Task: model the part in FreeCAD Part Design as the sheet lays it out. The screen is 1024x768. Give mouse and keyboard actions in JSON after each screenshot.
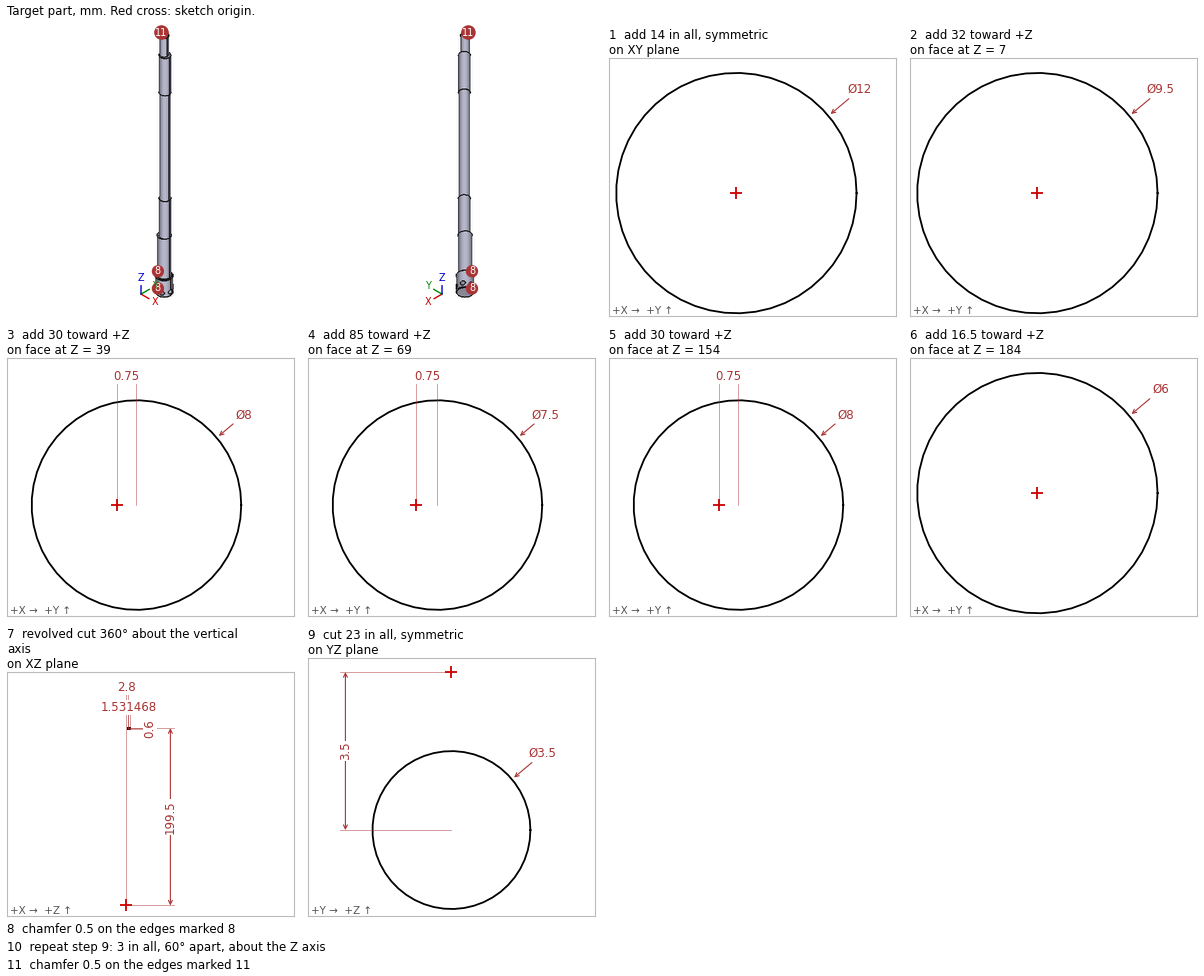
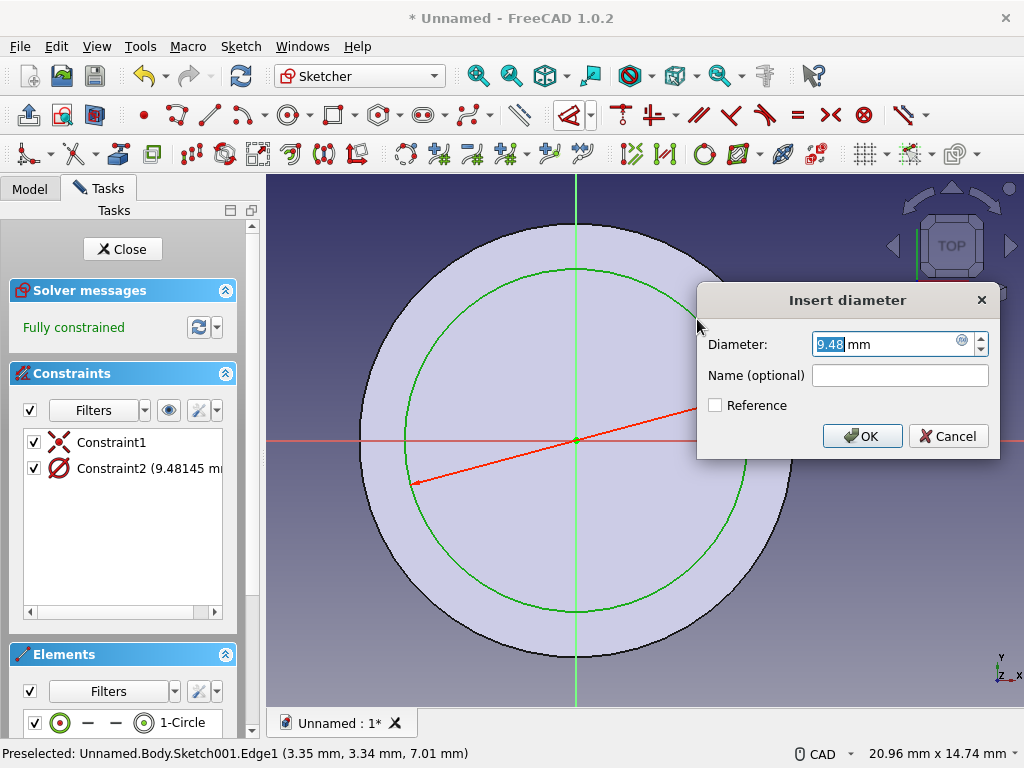
{"action": "type", "text": "9.5"}
{"action": "key", "text": "Return"}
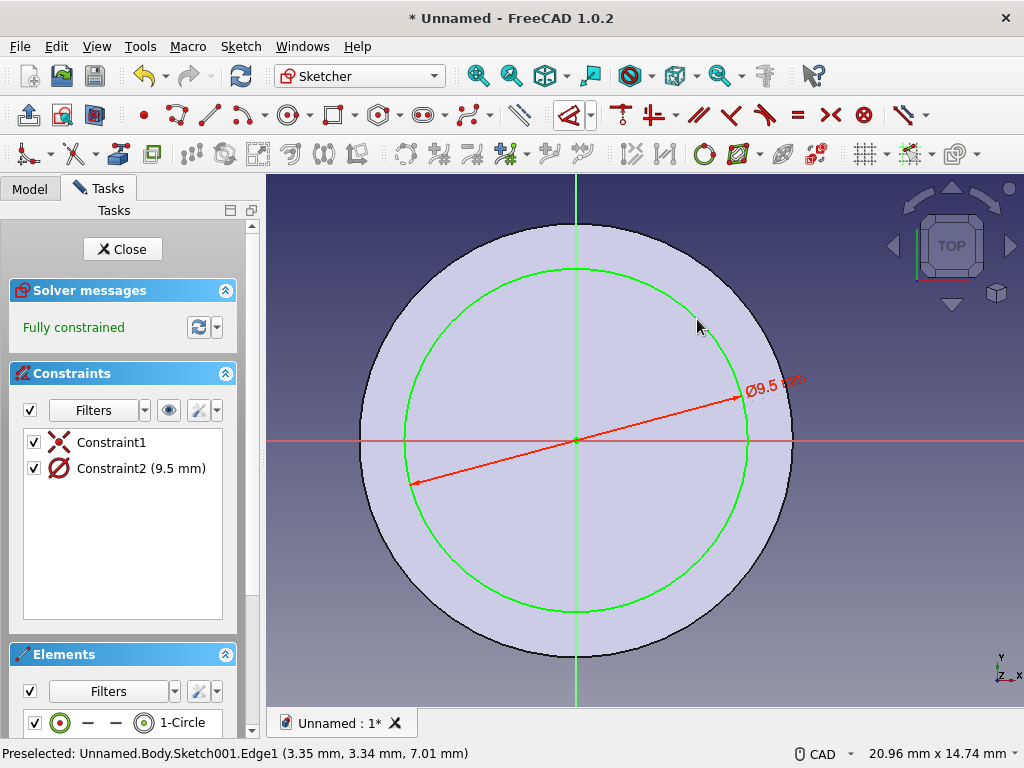
{"action": "left_click", "coordinate": [123, 249]}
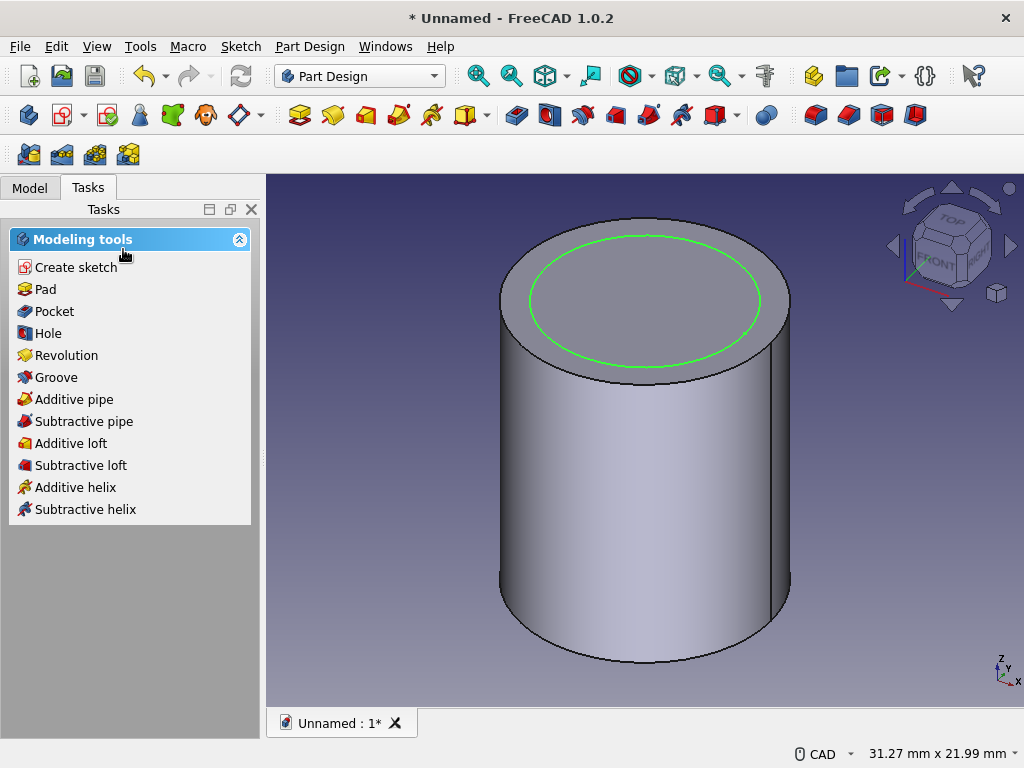
{"action": "left_click", "coordinate": [300, 116]}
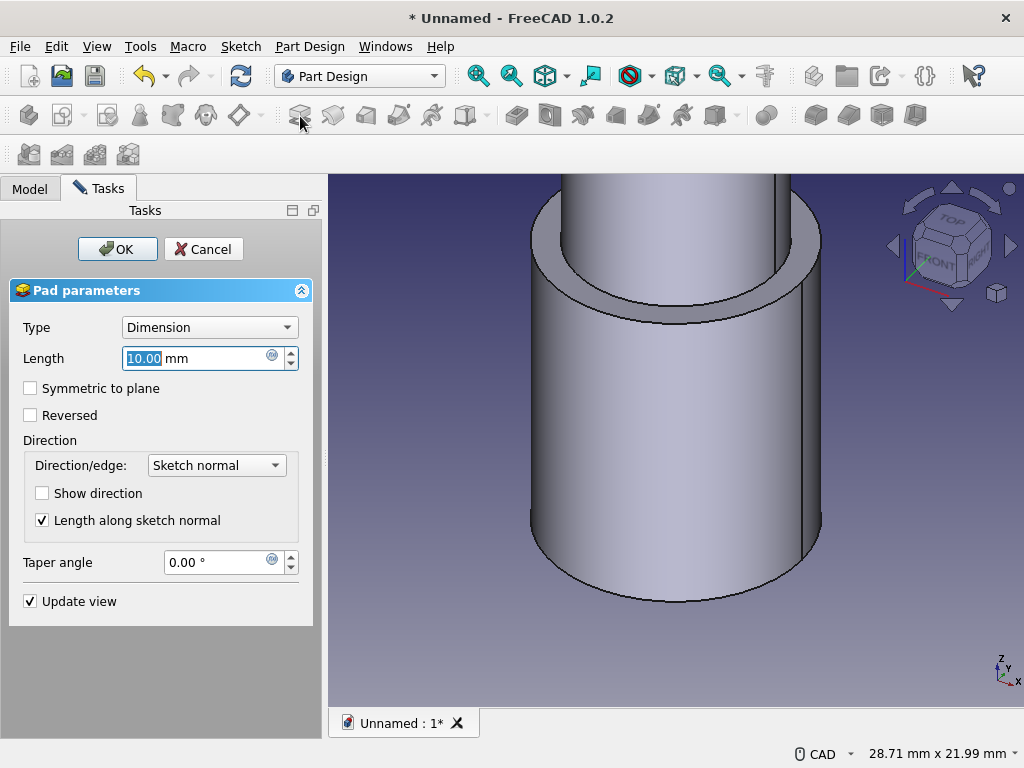
{"action": "type", "text": "32"}
{"action": "key", "text": "Tab"}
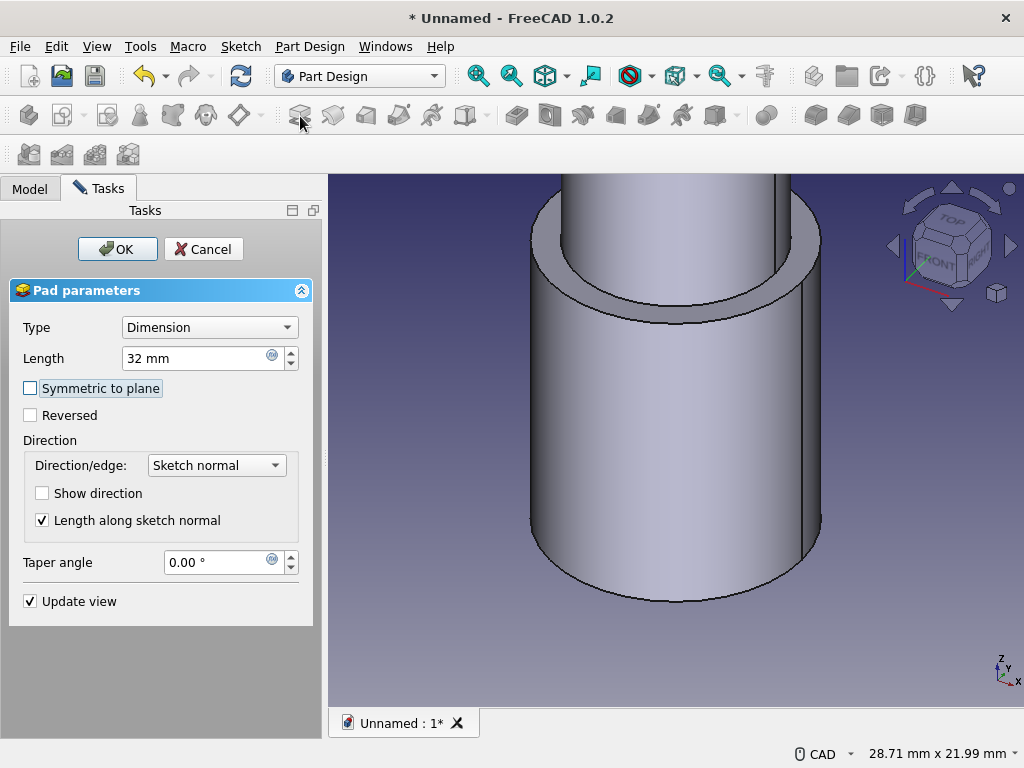
{"action": "left_click", "coordinate": [118, 249]}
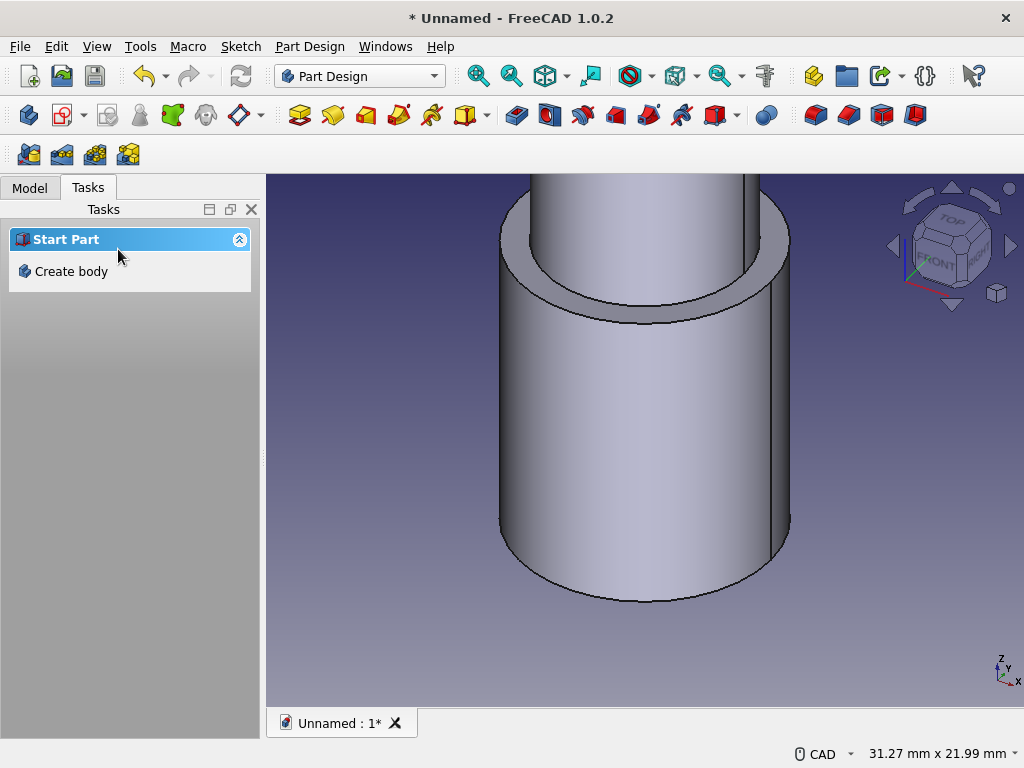
{"action": "key", "text": "v f"}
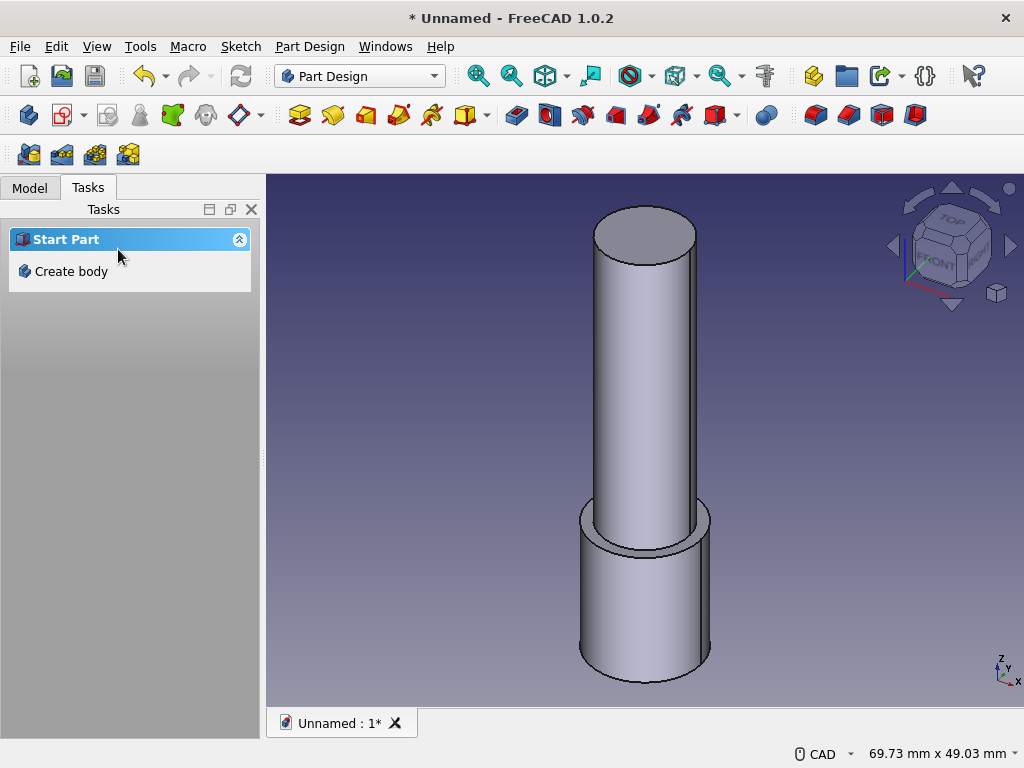
{"action": "left_click", "coordinate": [645, 235]}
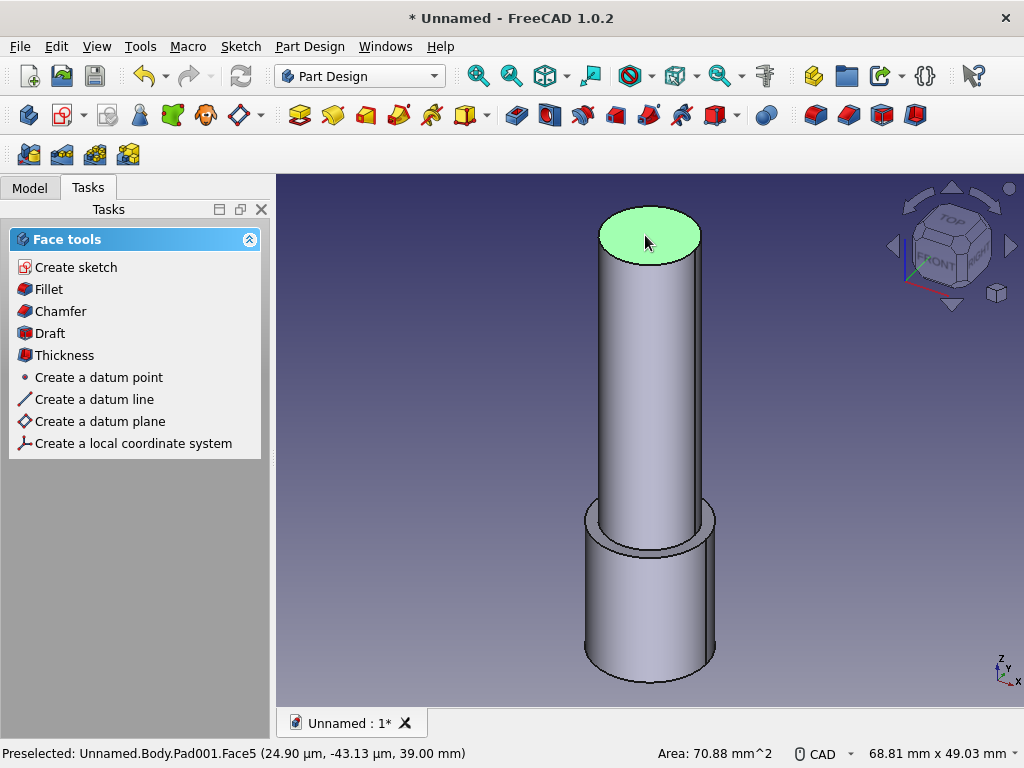
{"action": "left_click", "coordinate": [62, 116]}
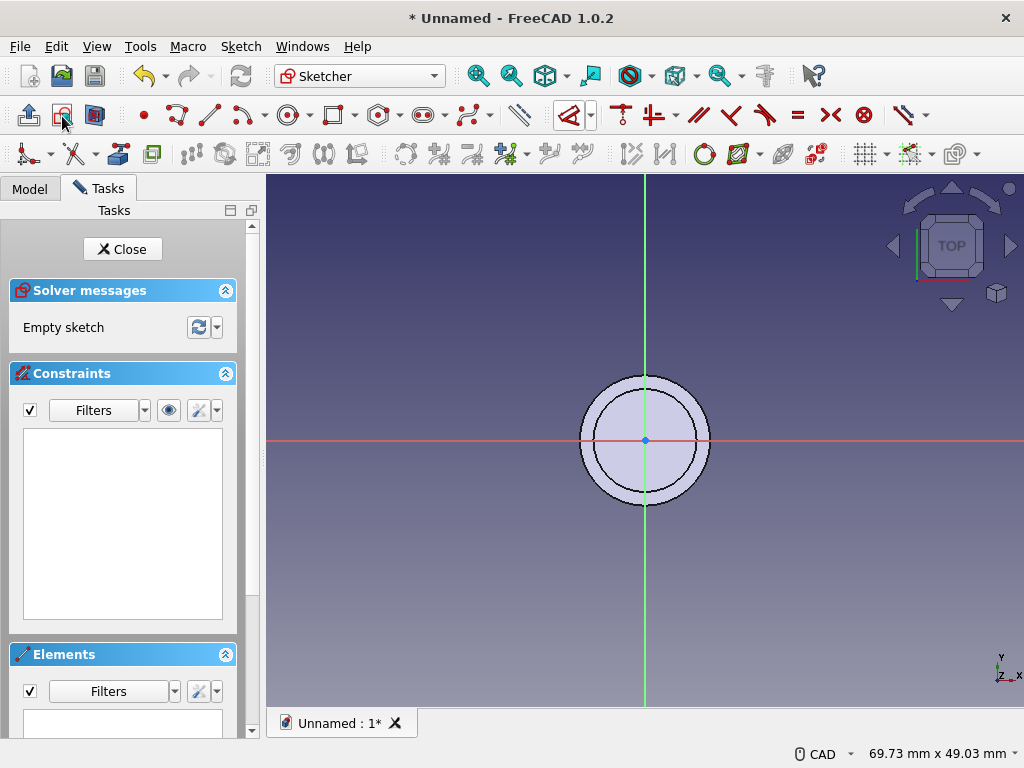
{"action": "scroll", "coordinate": [678, 440], "scroll_direction": "up", "scroll_amount": 7}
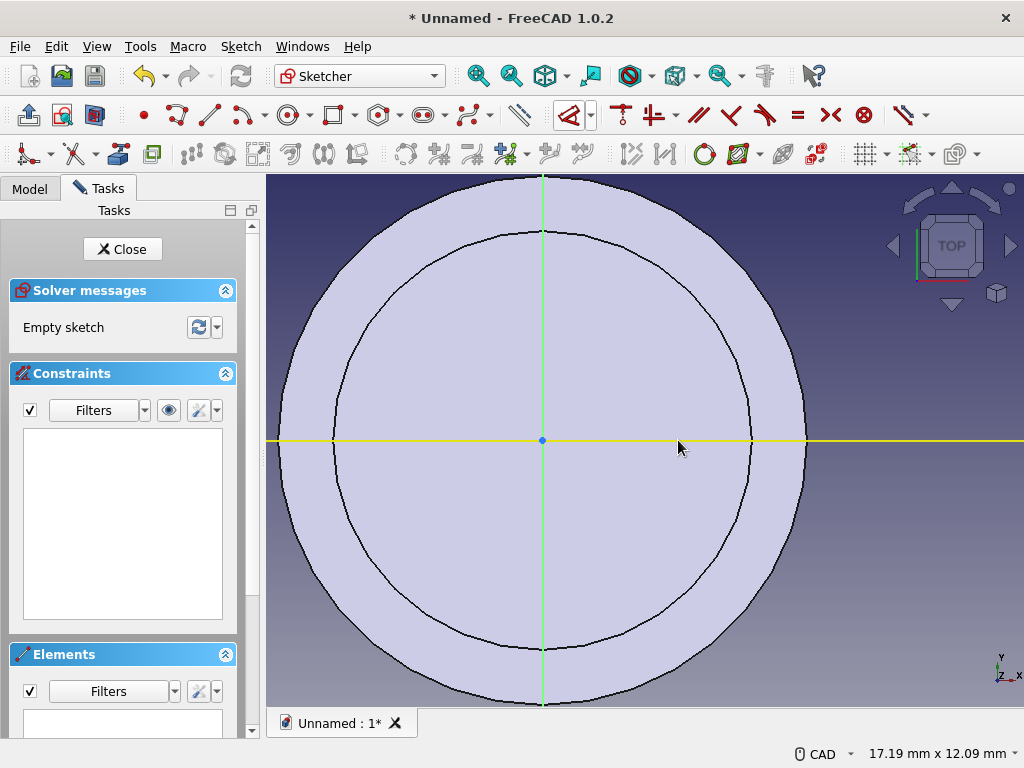
{"action": "key", "text": "g c"}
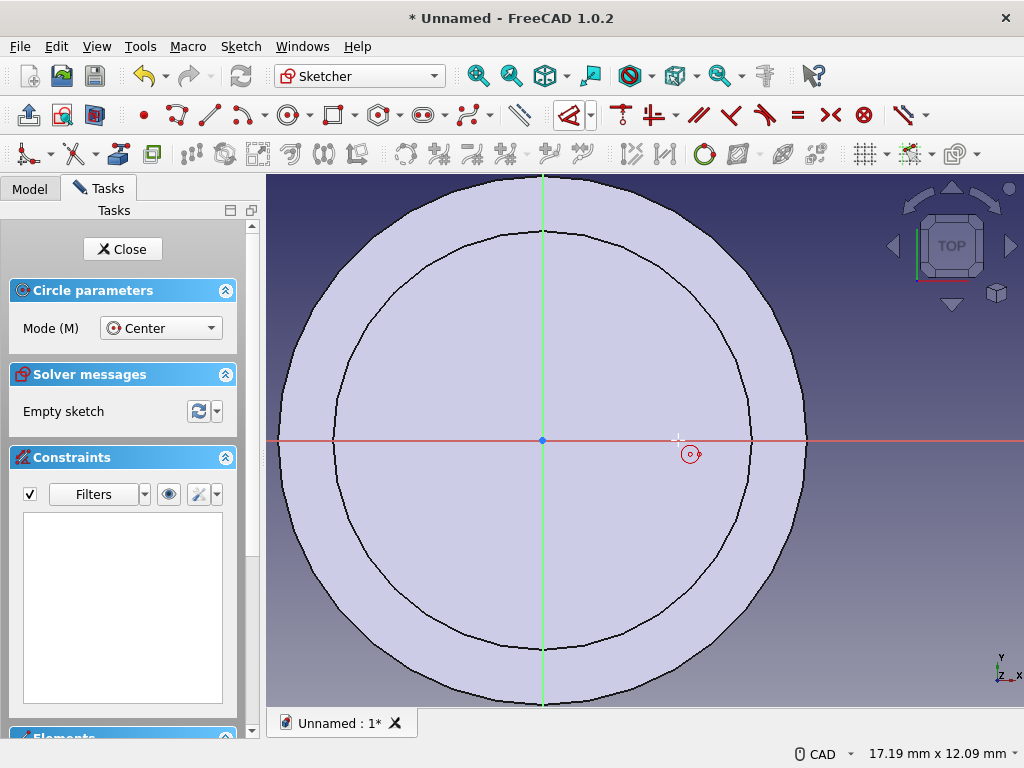
{"action": "left_click", "coordinate": [576, 440]}
{"action": "left_click", "coordinate": [700, 316]}
{"action": "key", "text": "Escape"}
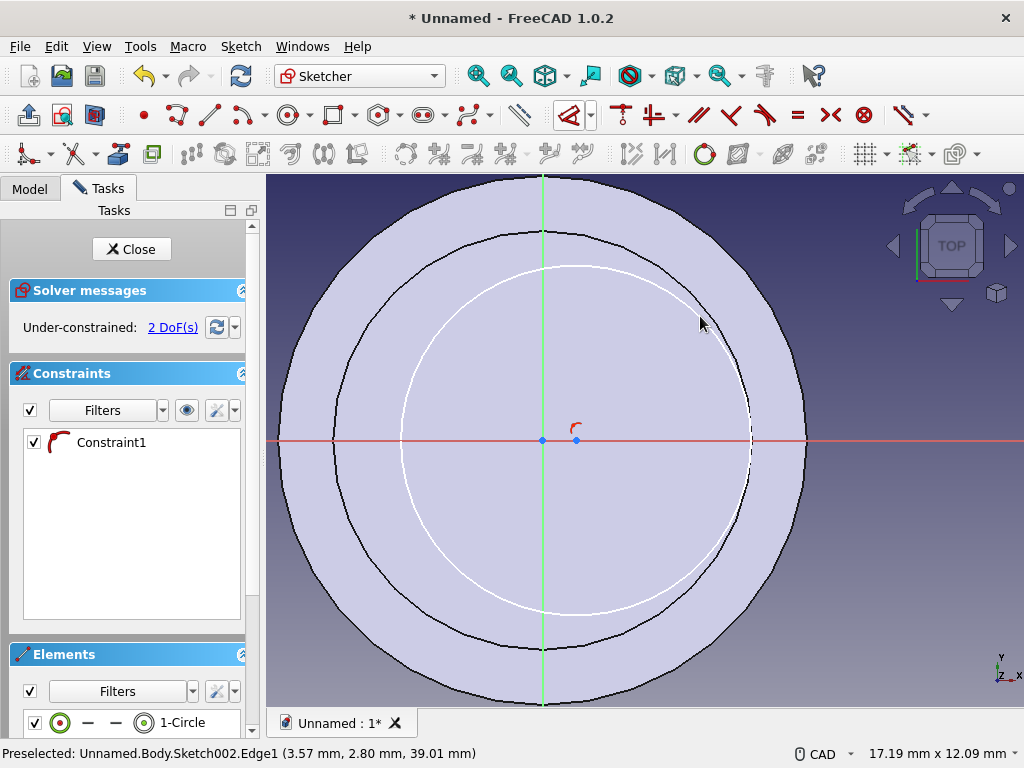
{"action": "left_click", "coordinate": [699, 316]}